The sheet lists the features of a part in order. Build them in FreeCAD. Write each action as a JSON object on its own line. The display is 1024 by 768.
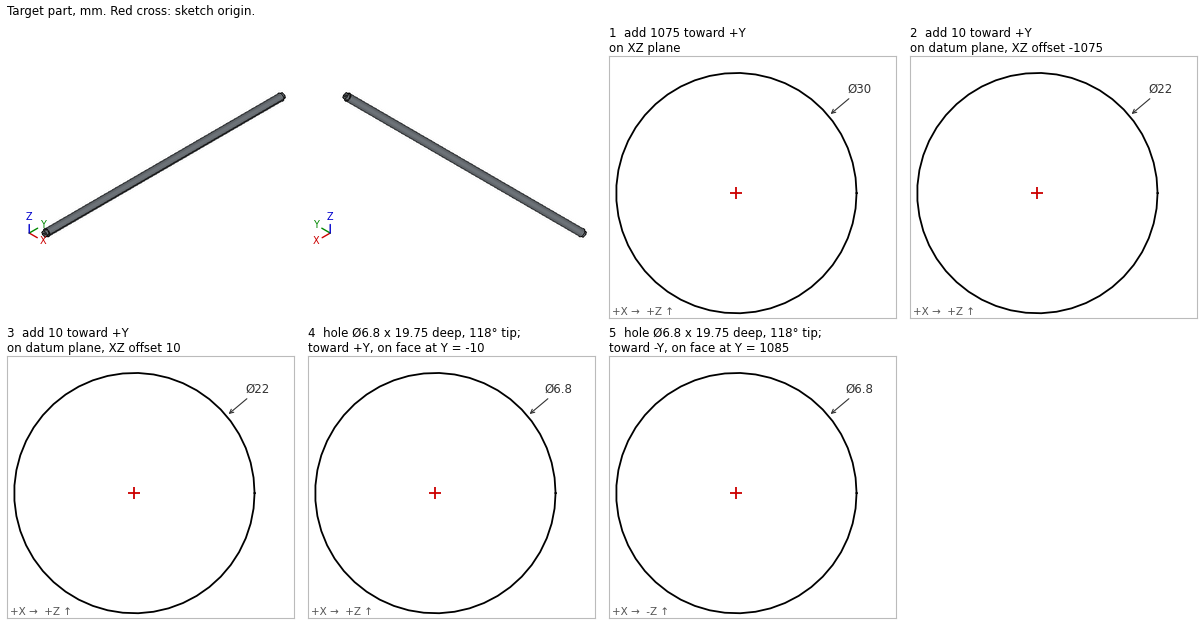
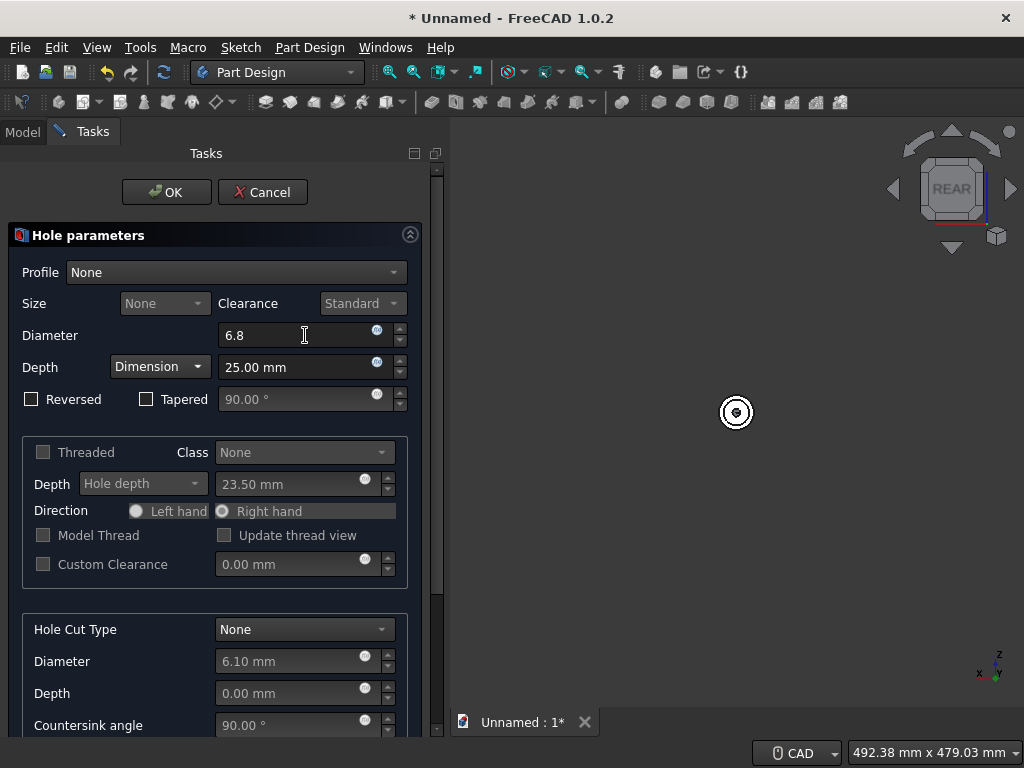
{"action": "triple_click", "coordinate": [305, 367]}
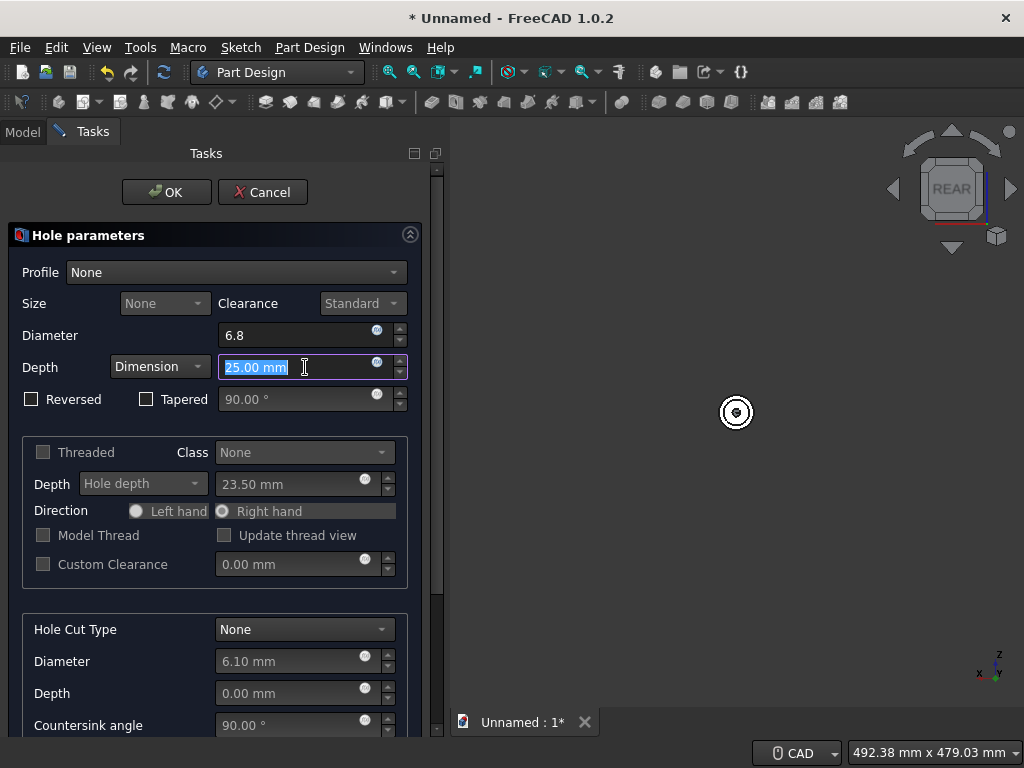
{"action": "type", "text": "19.75"}
{"action": "key", "text": "Tab"}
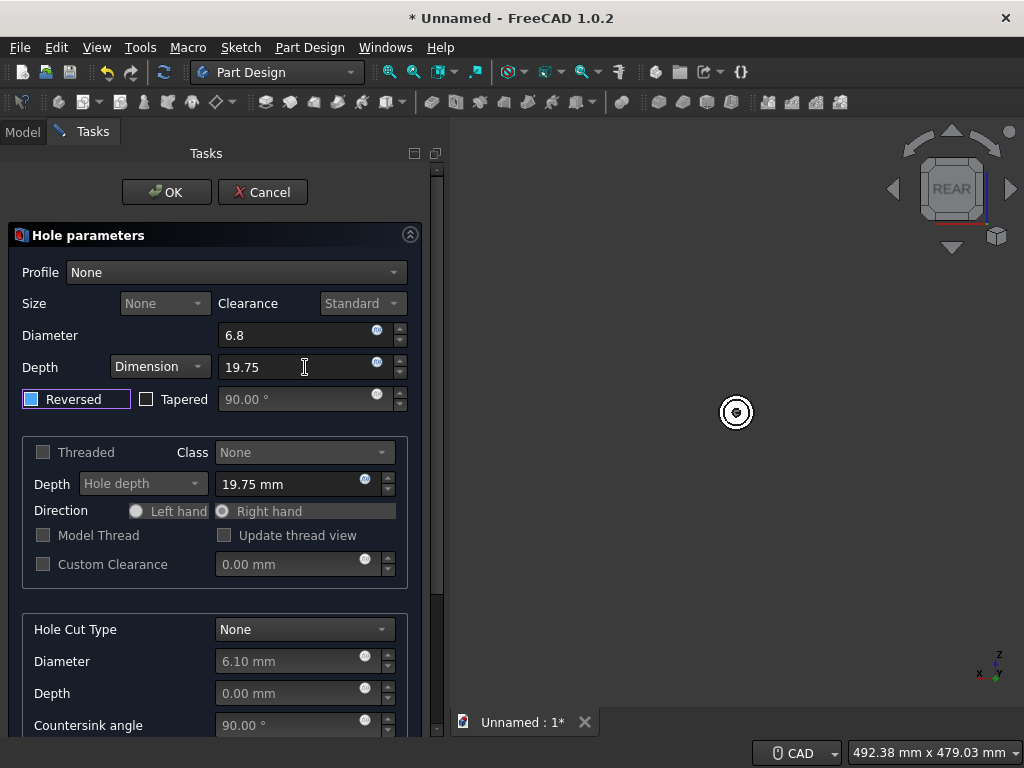
{"action": "left_click", "coordinate": [167, 192]}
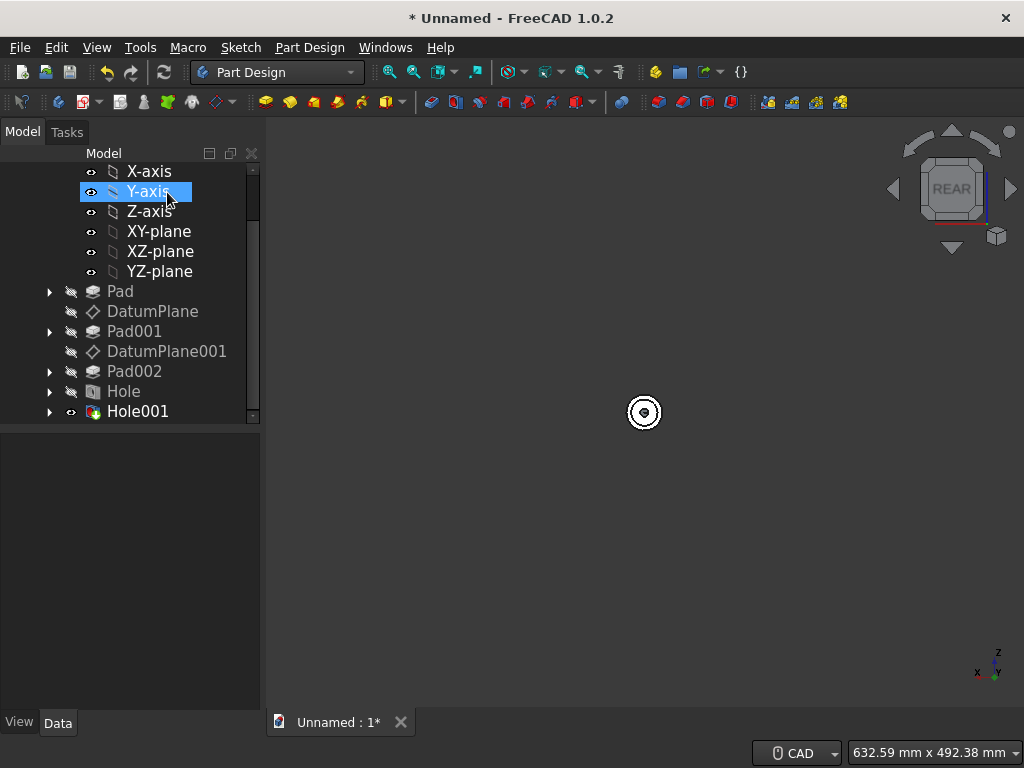
{"action": "key", "text": "0"}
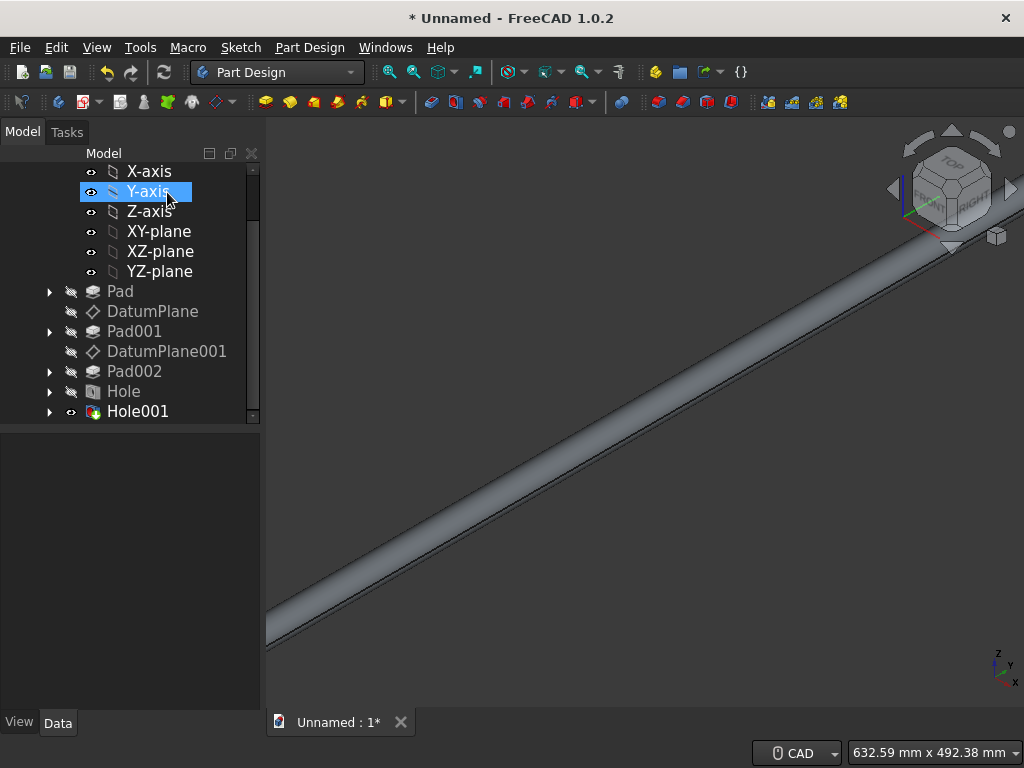
{"action": "left_click", "coordinate": [390, 72]}